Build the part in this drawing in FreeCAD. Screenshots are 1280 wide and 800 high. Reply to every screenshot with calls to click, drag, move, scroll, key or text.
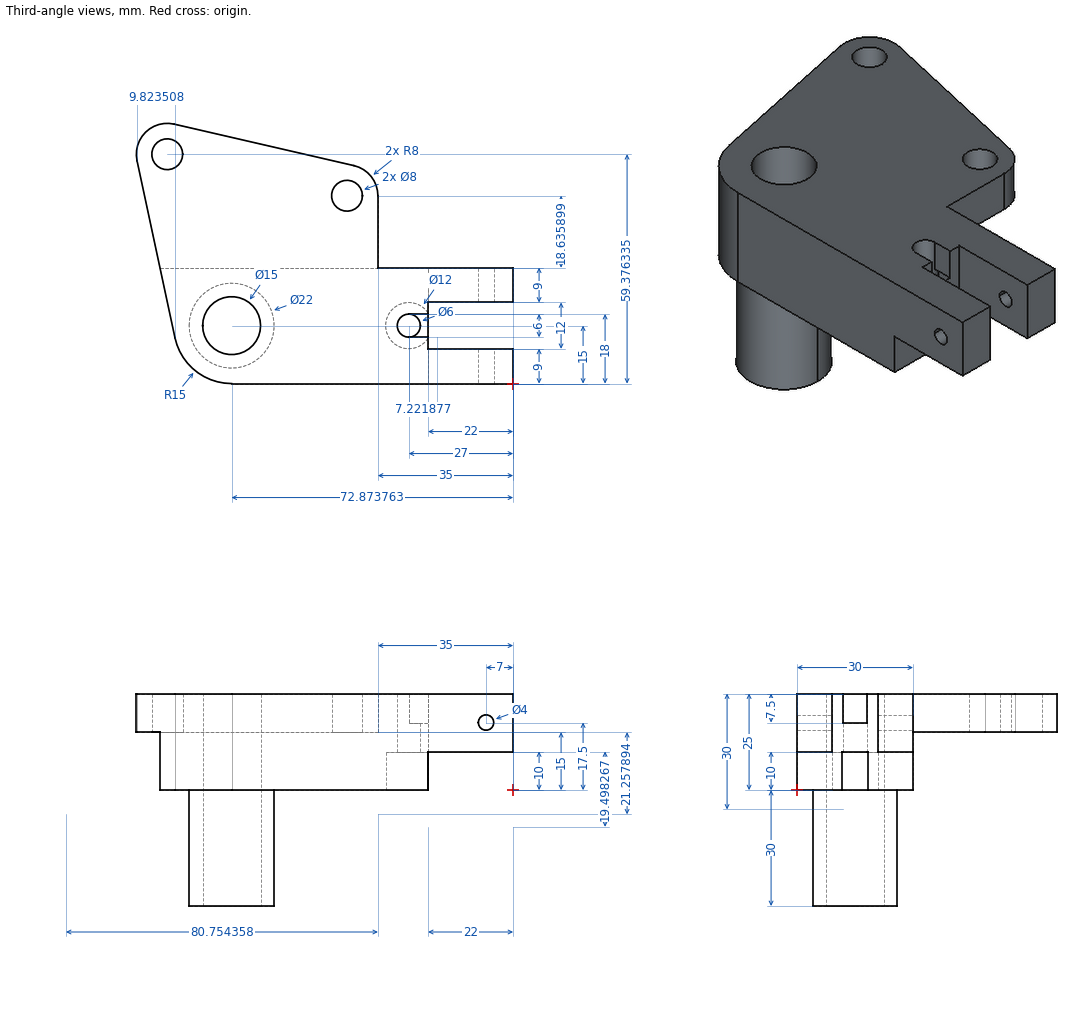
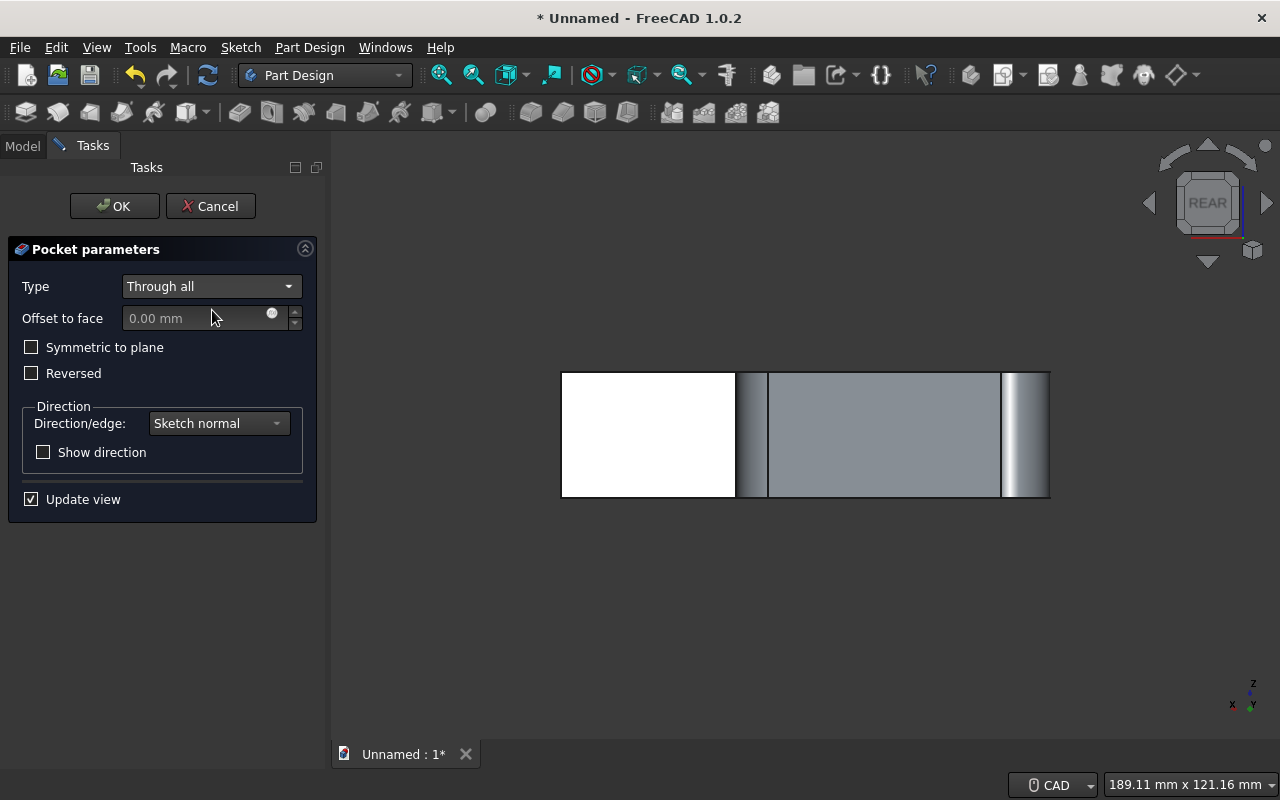
click(30, 373)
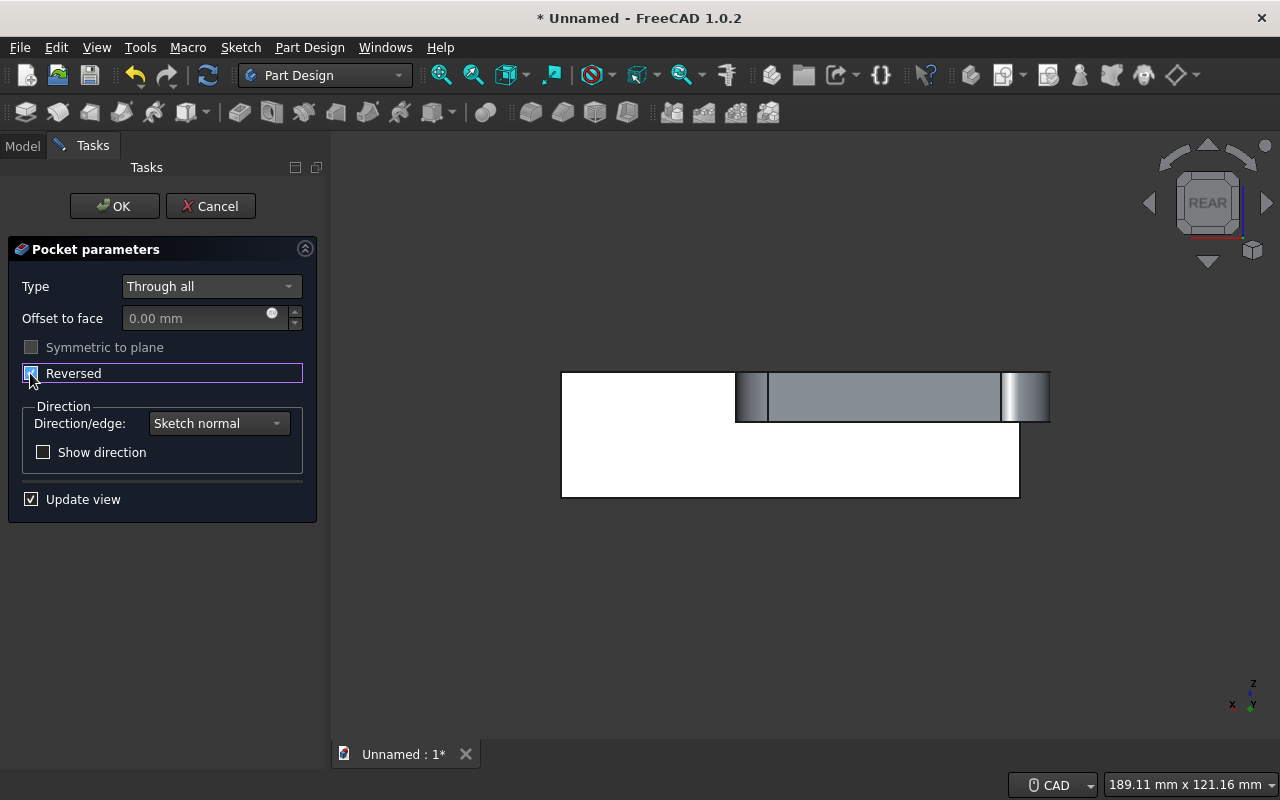
click(115, 206)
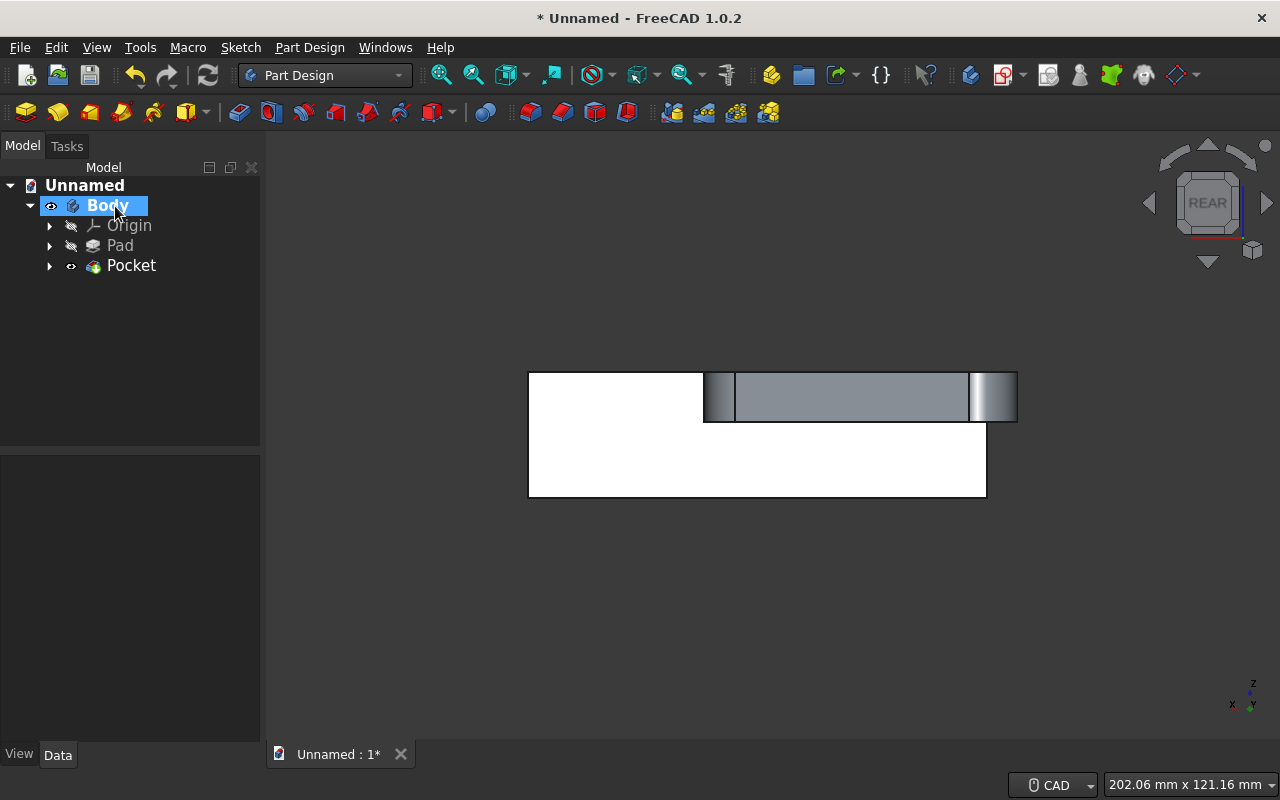
click(1004, 76)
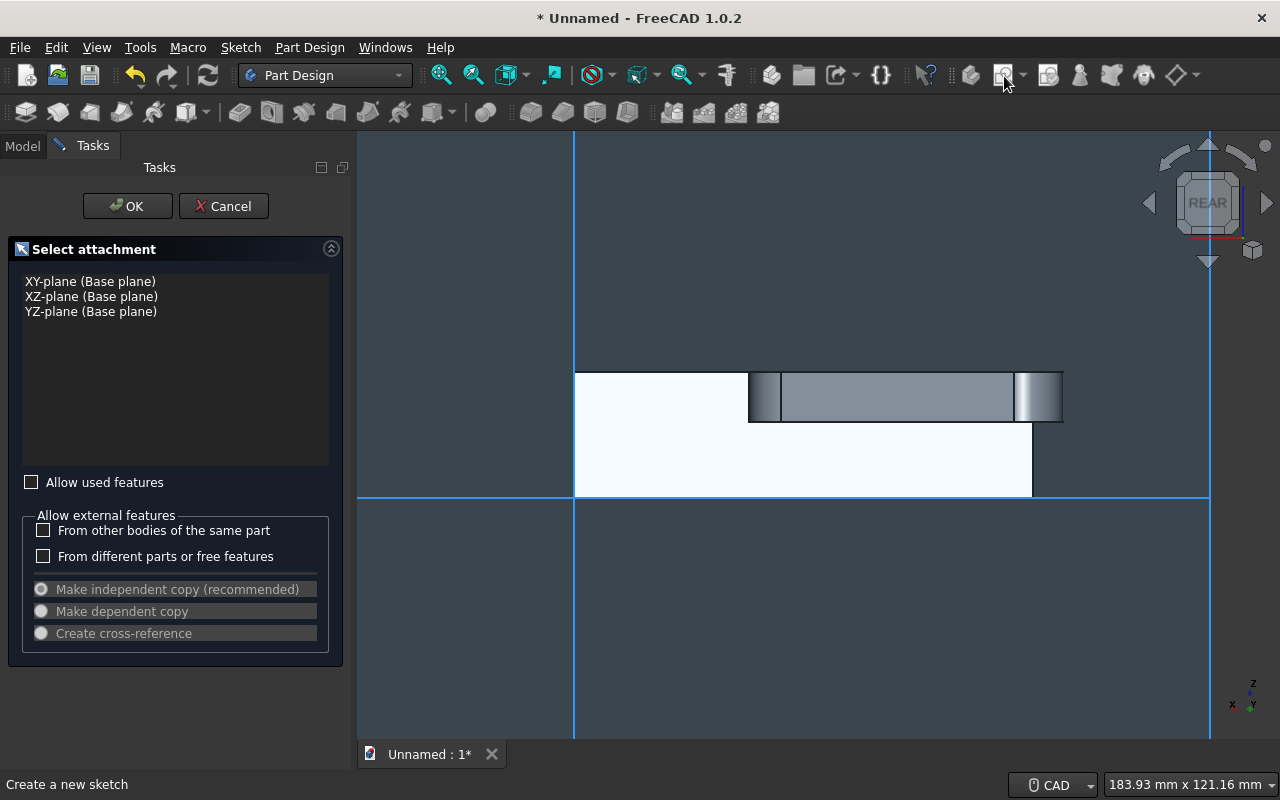
click(82, 282)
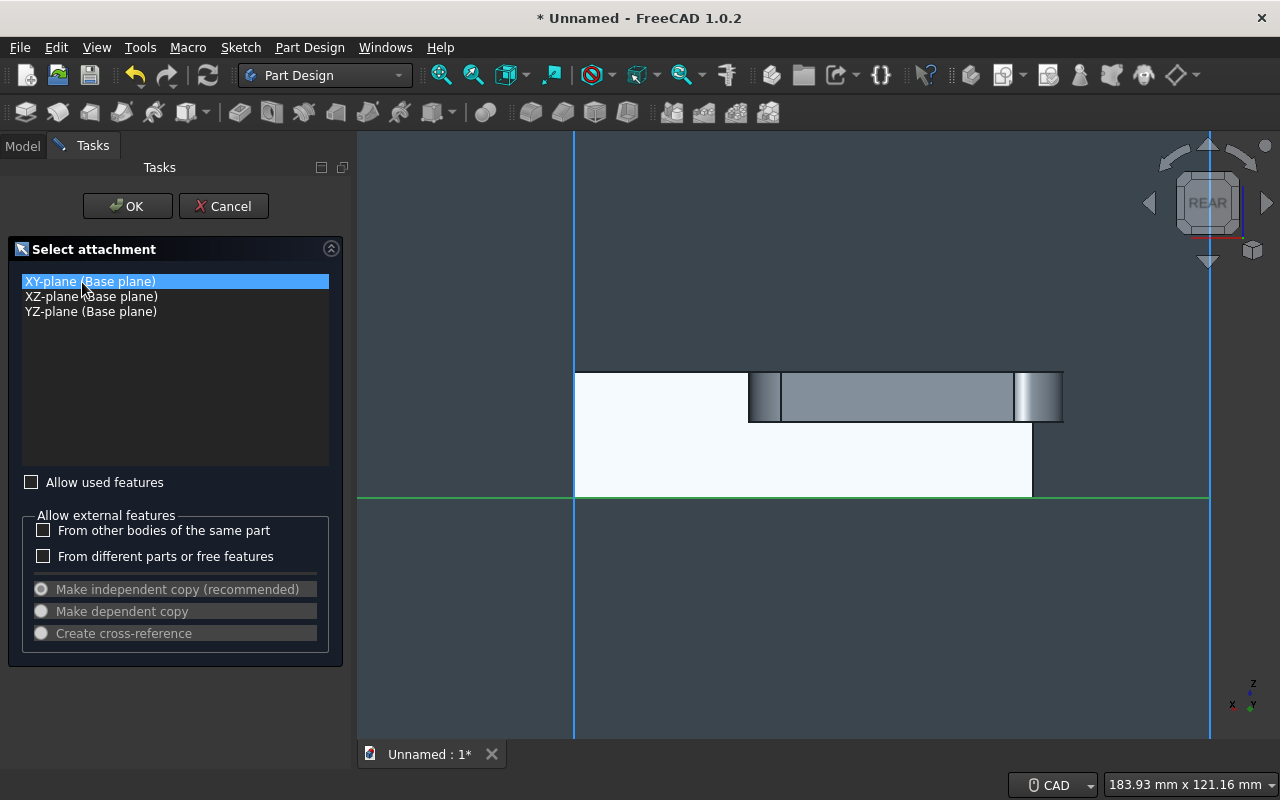
click(128, 206)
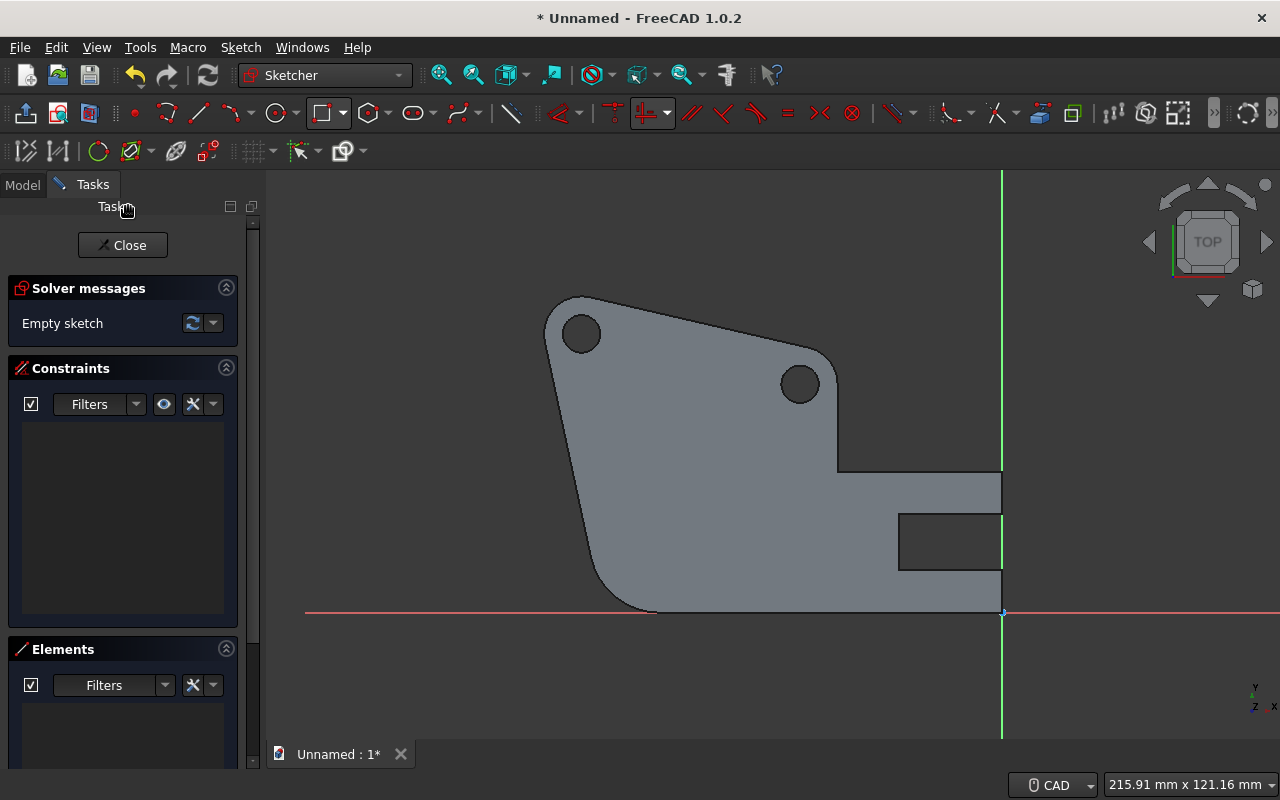
click(90, 114)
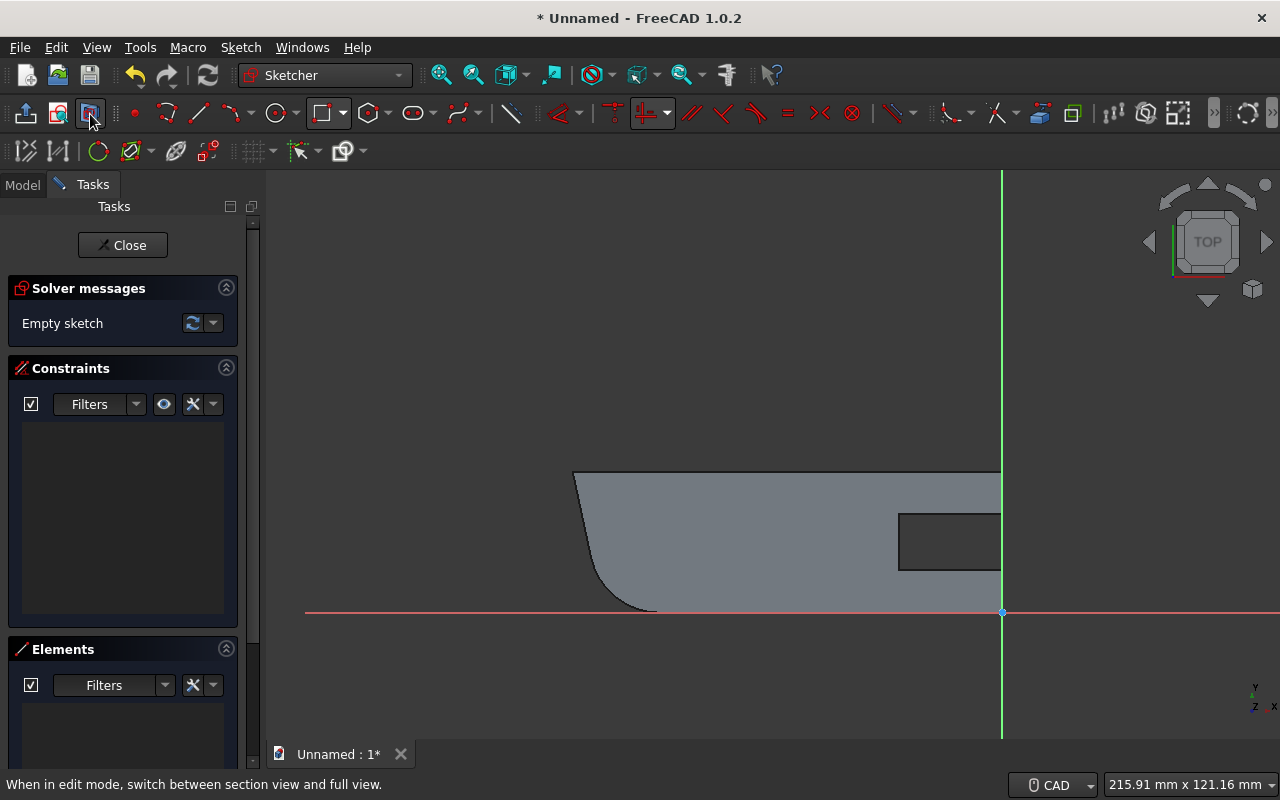
scroll(641, 580, up, 6)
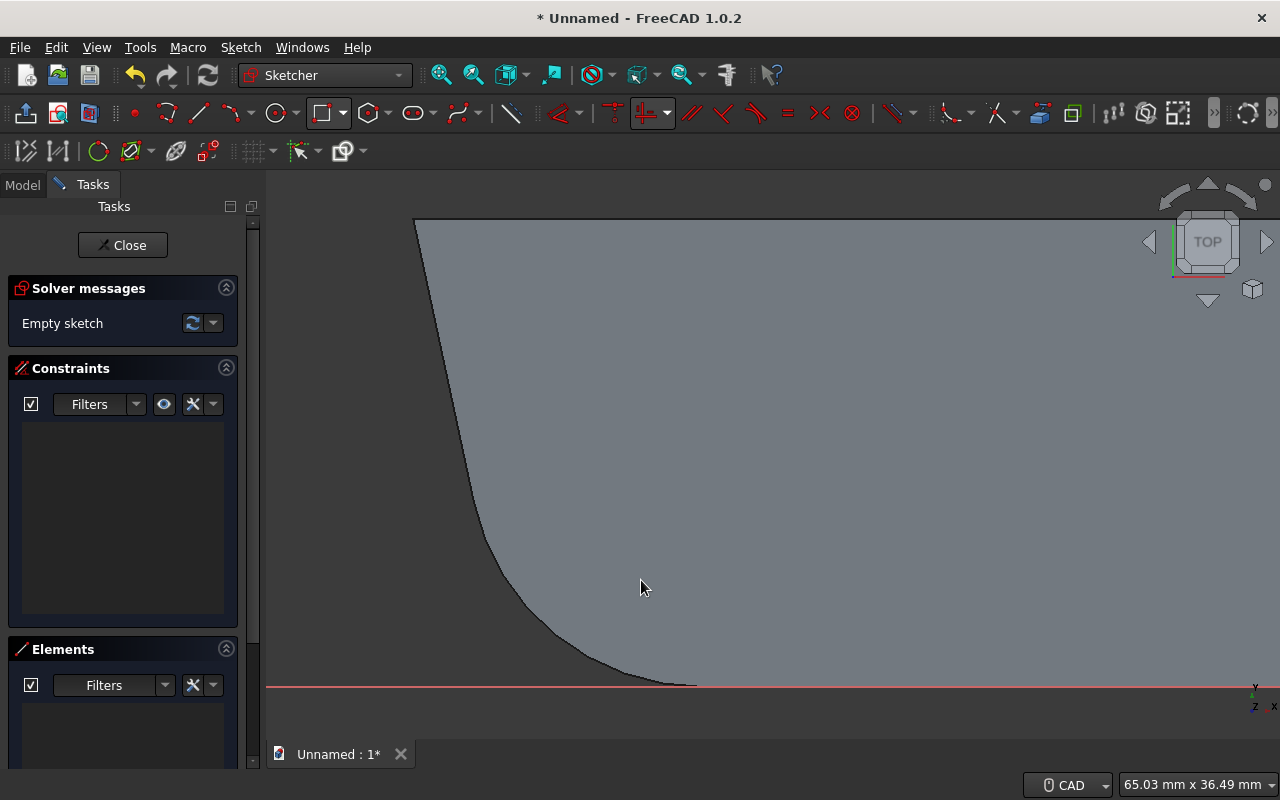
click(276, 114)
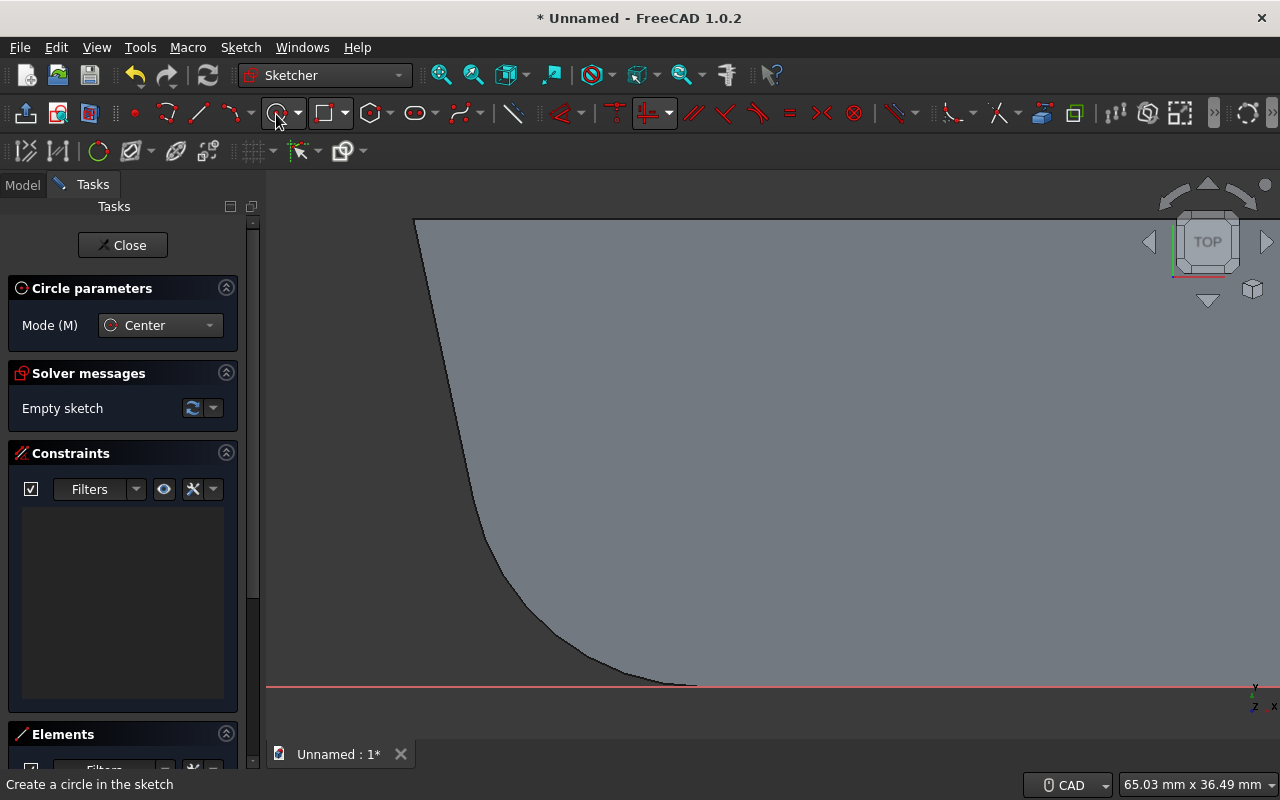
click(703, 453)
click(824, 332)
key(Escape)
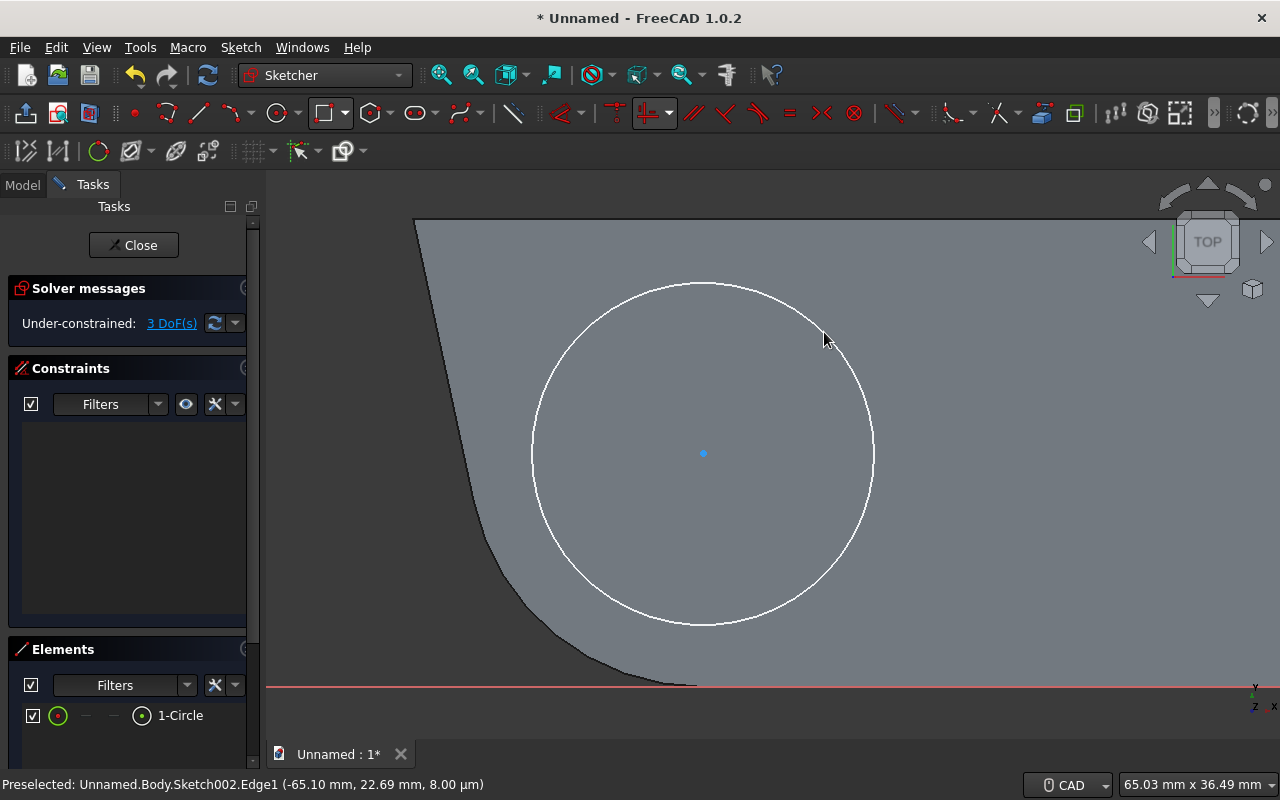
click(560, 114)